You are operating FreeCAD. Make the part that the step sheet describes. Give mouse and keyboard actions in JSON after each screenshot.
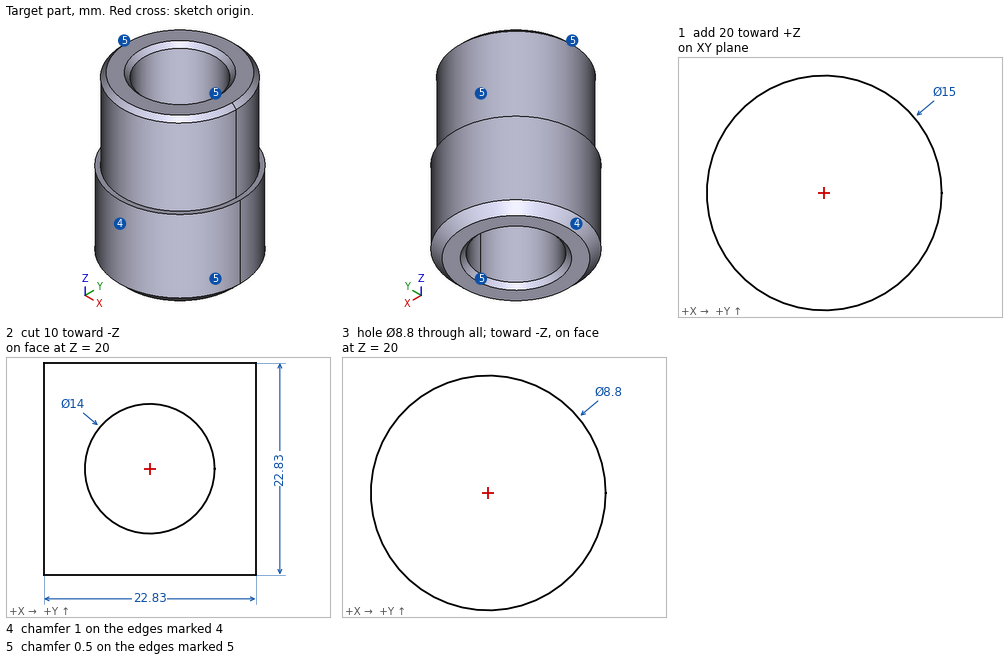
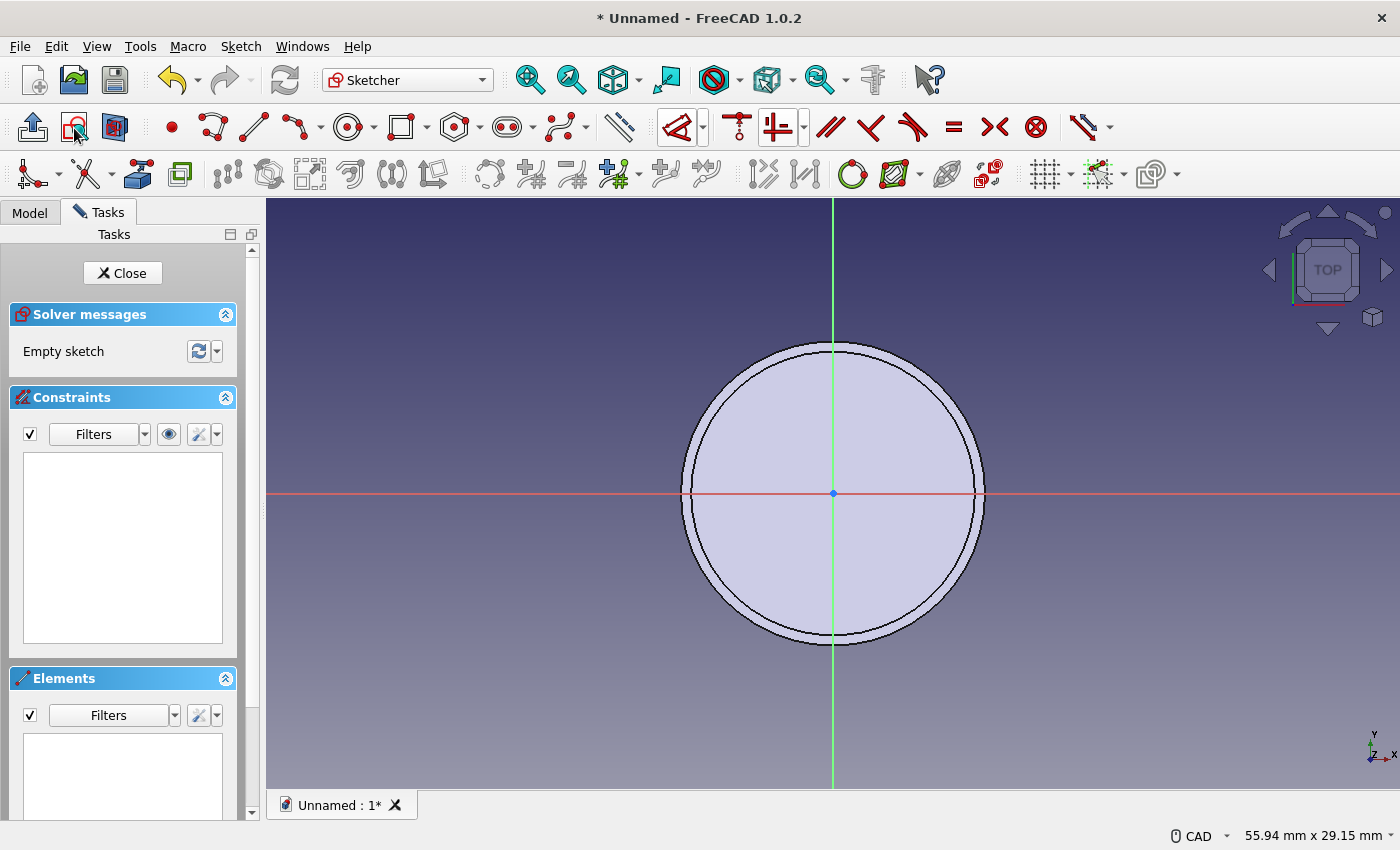
{"action": "scroll", "coordinate": [889, 494], "scroll_direction": "up", "scroll_amount": 4}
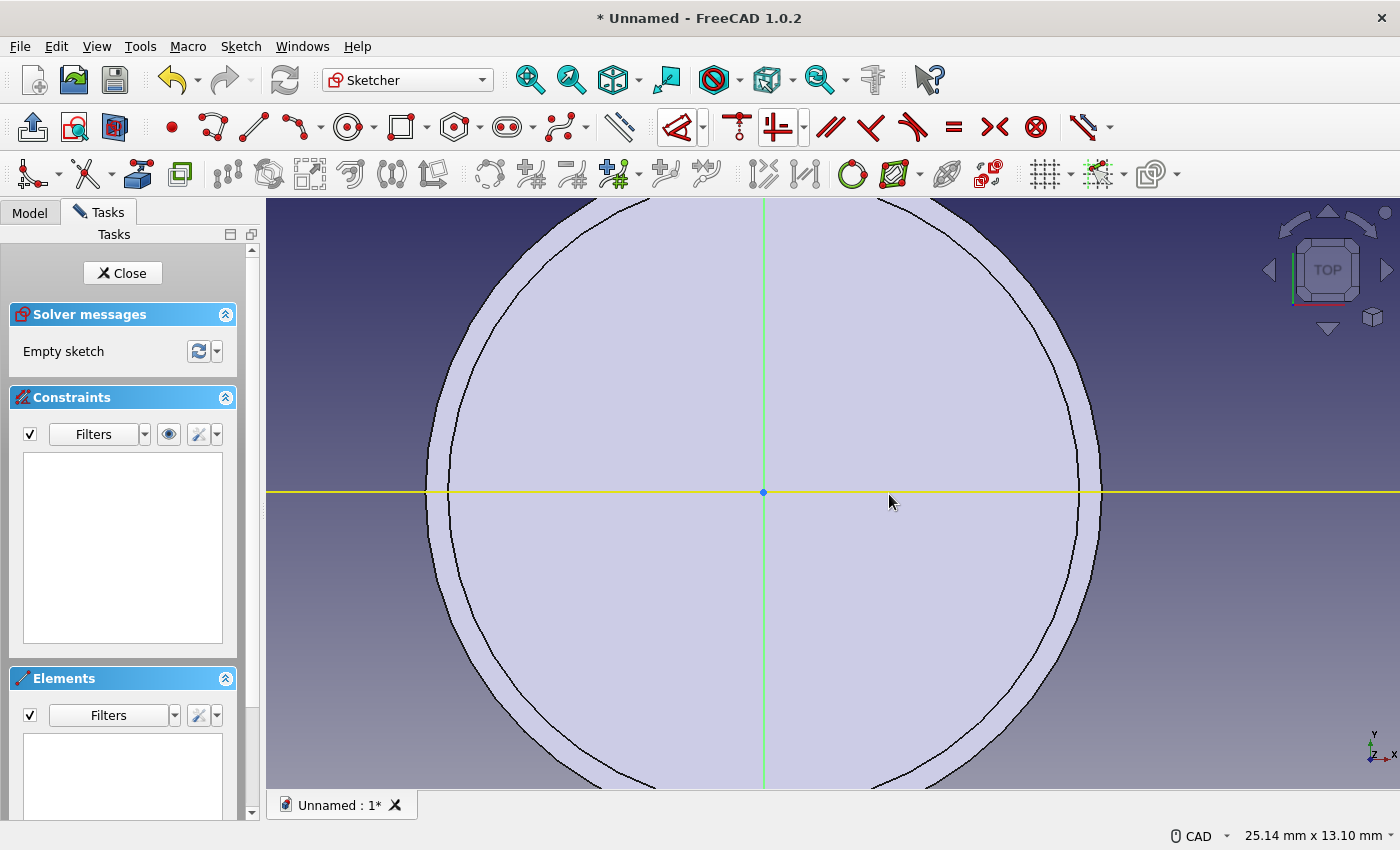
{"action": "left_click", "coordinate": [348, 128]}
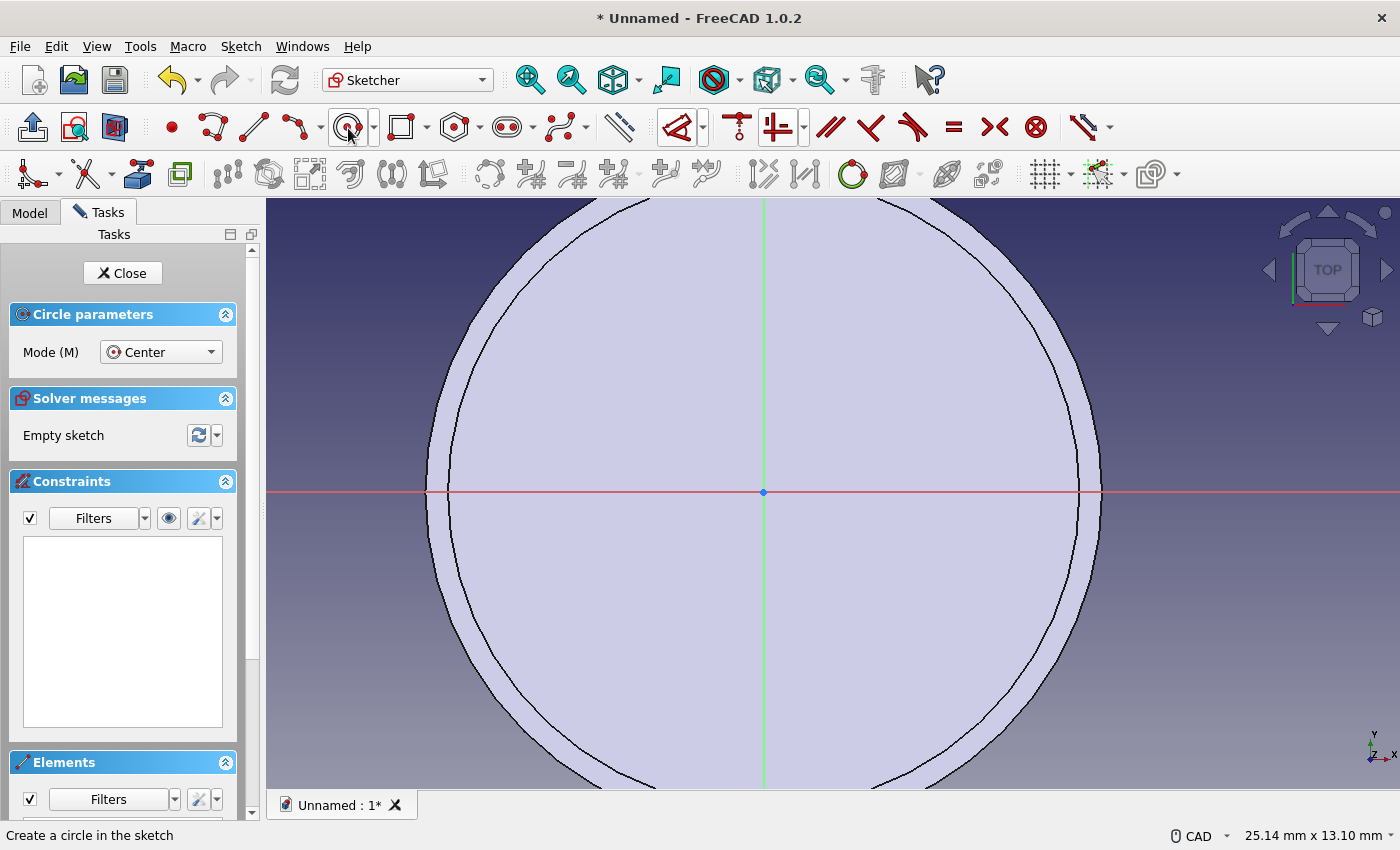
{"action": "left_click", "coordinate": [764, 492]}
{"action": "mouse_move", "coordinate": [904, 352]}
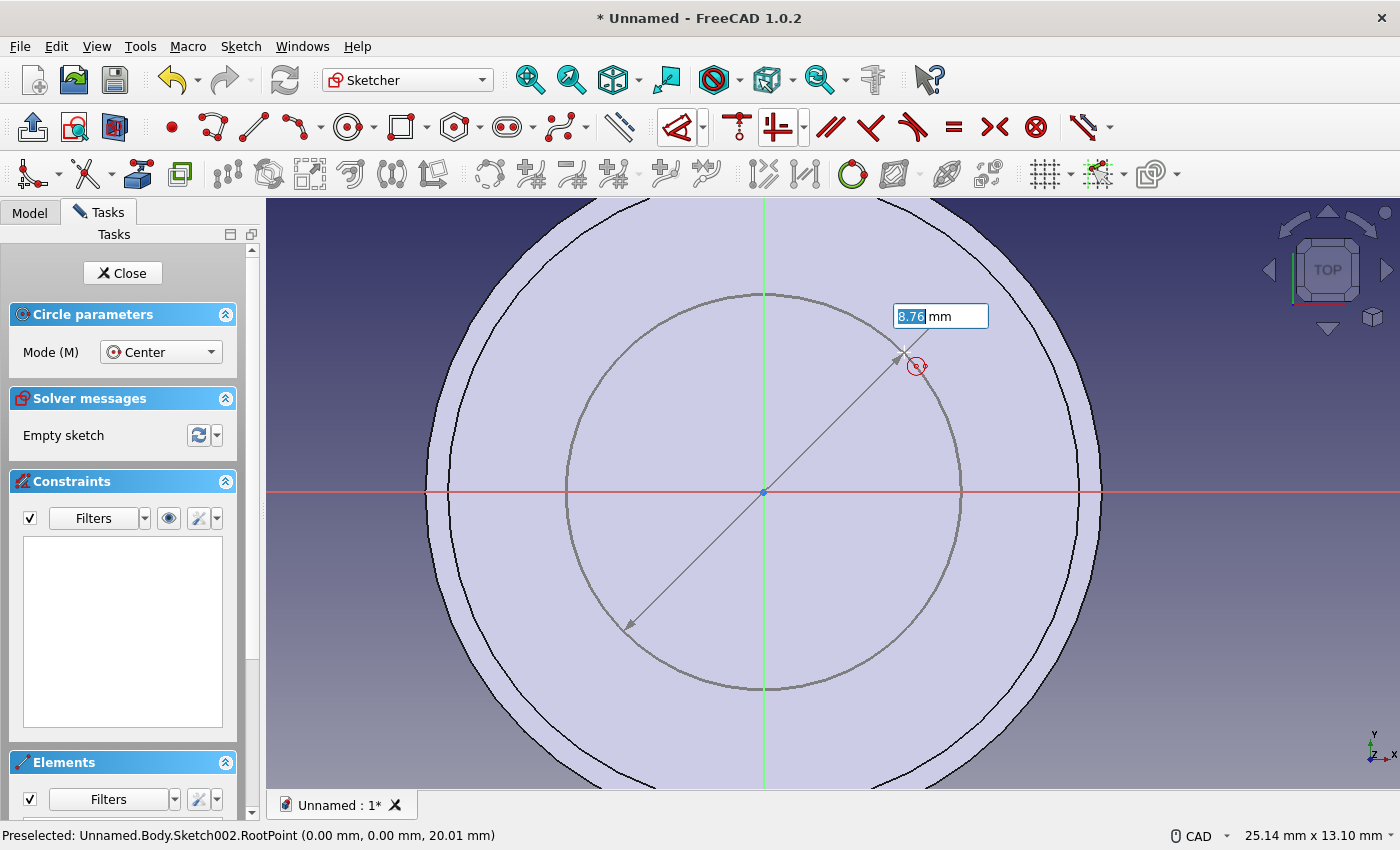
{"action": "type", "text": "8.8"}
{"action": "key", "text": "Return"}
{"action": "key", "text": "Escape"}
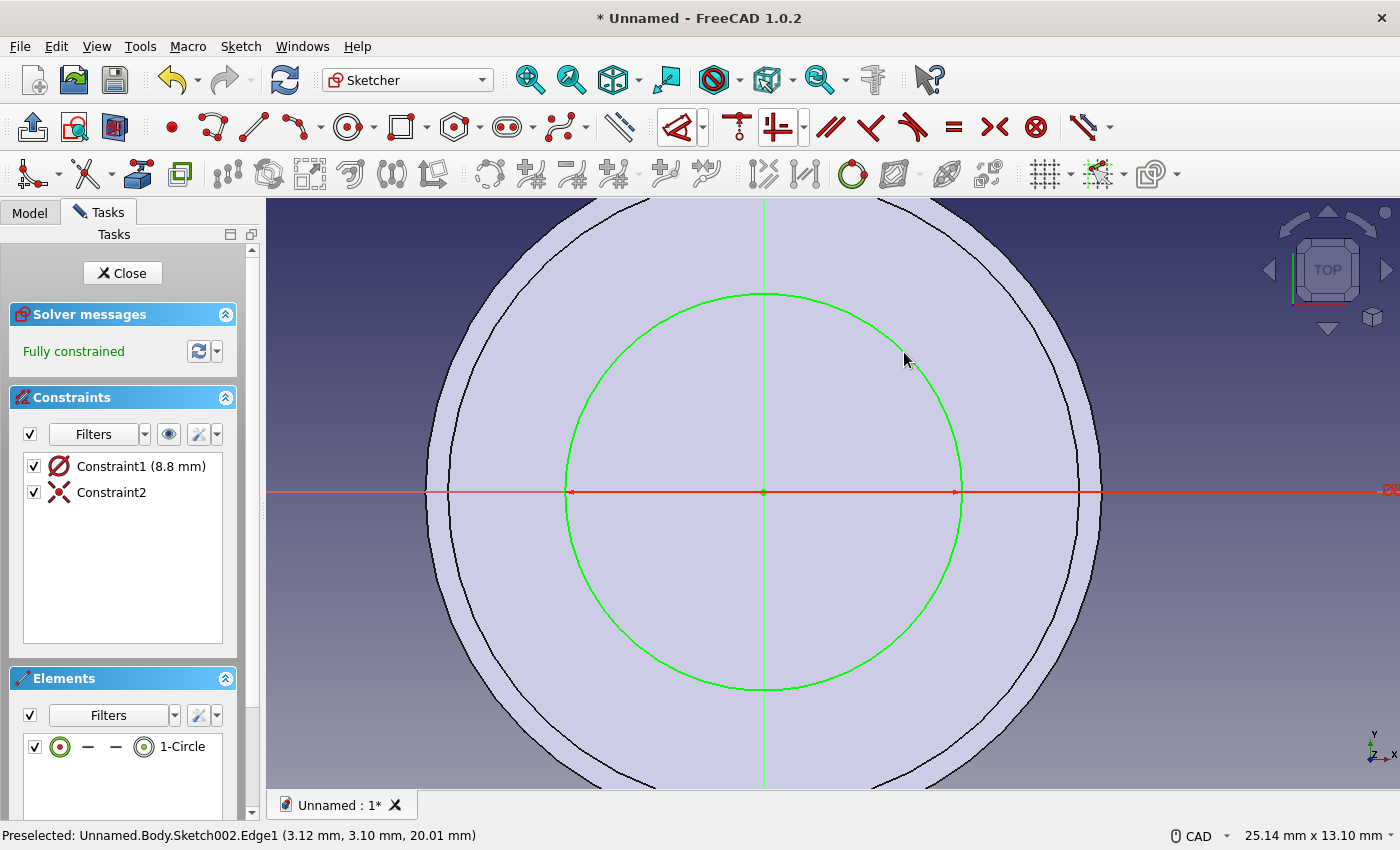
{"action": "left_click", "coordinate": [123, 273]}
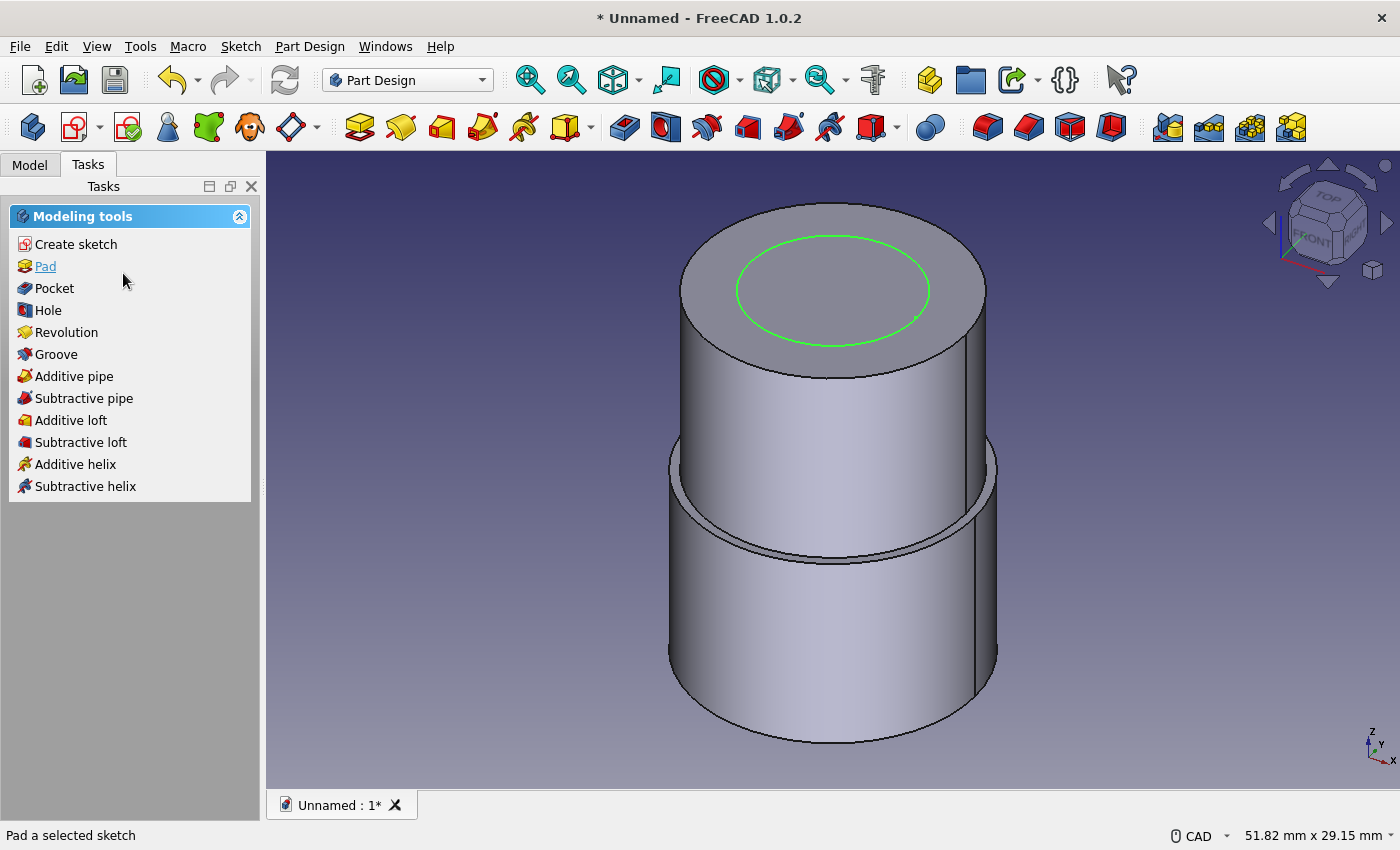
{"action": "left_click", "coordinate": [666, 128]}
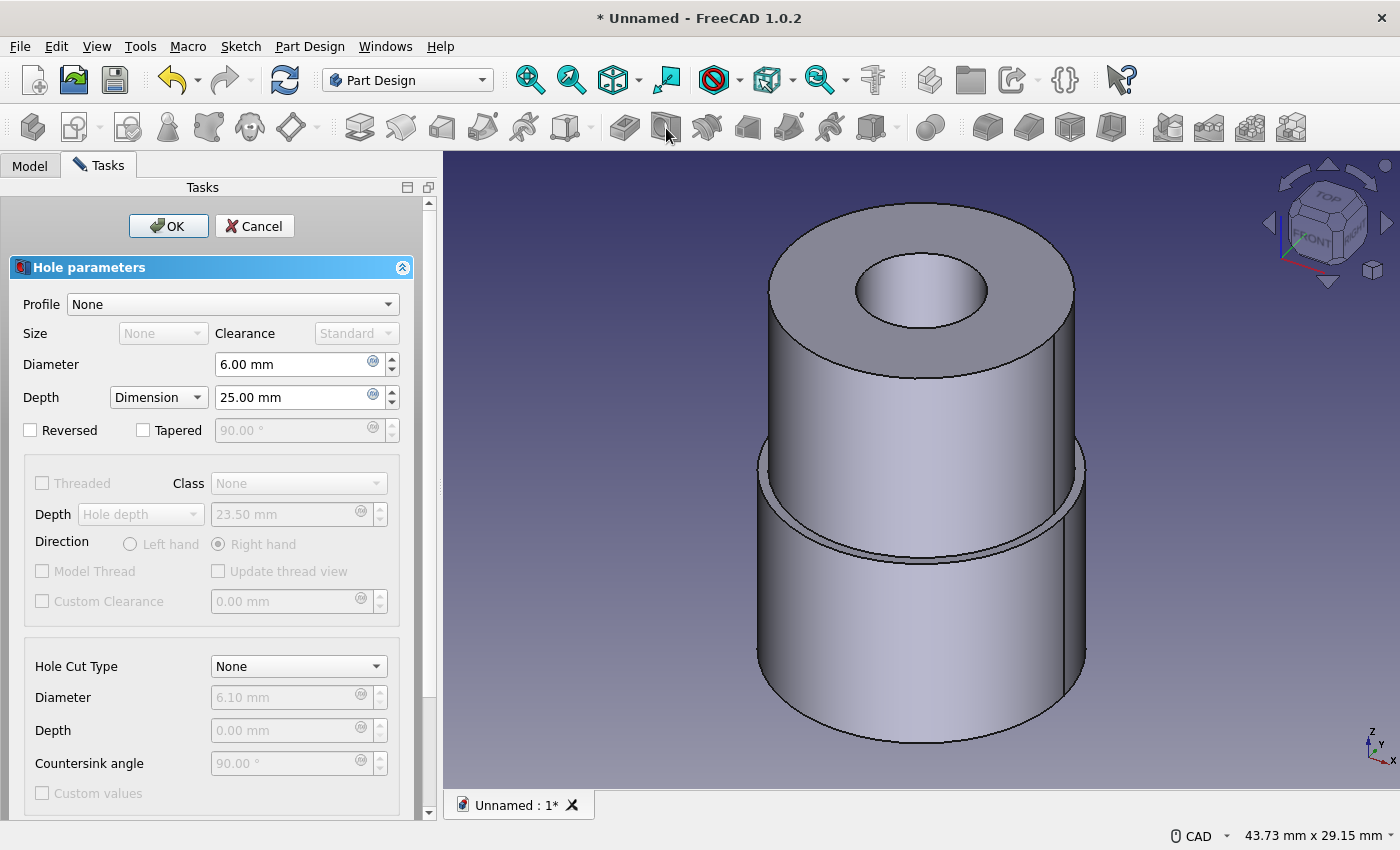
{"action": "triple_click", "coordinate": [300, 364]}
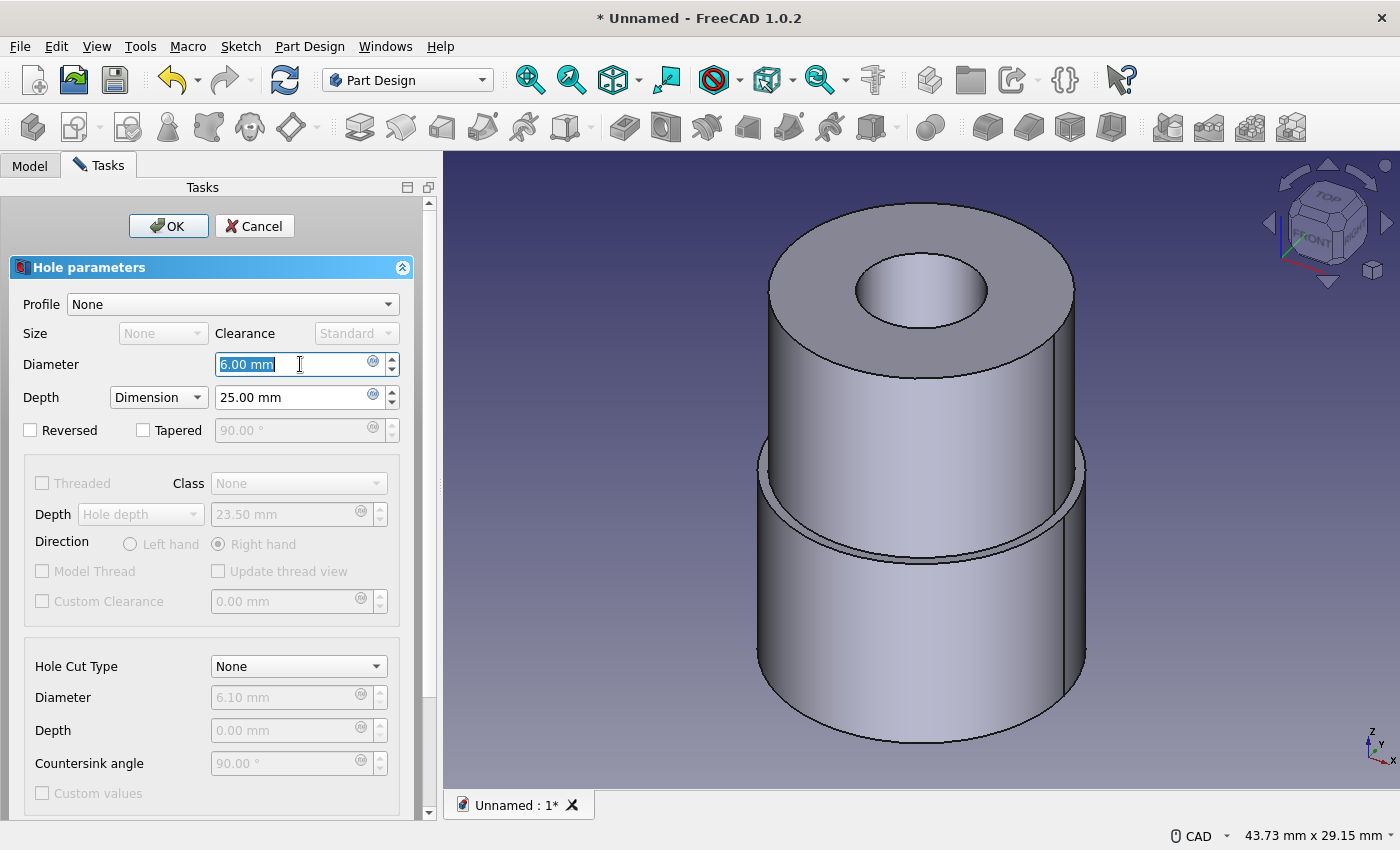
{"action": "type", "text": "8.8"}
{"action": "key", "text": "Tab"}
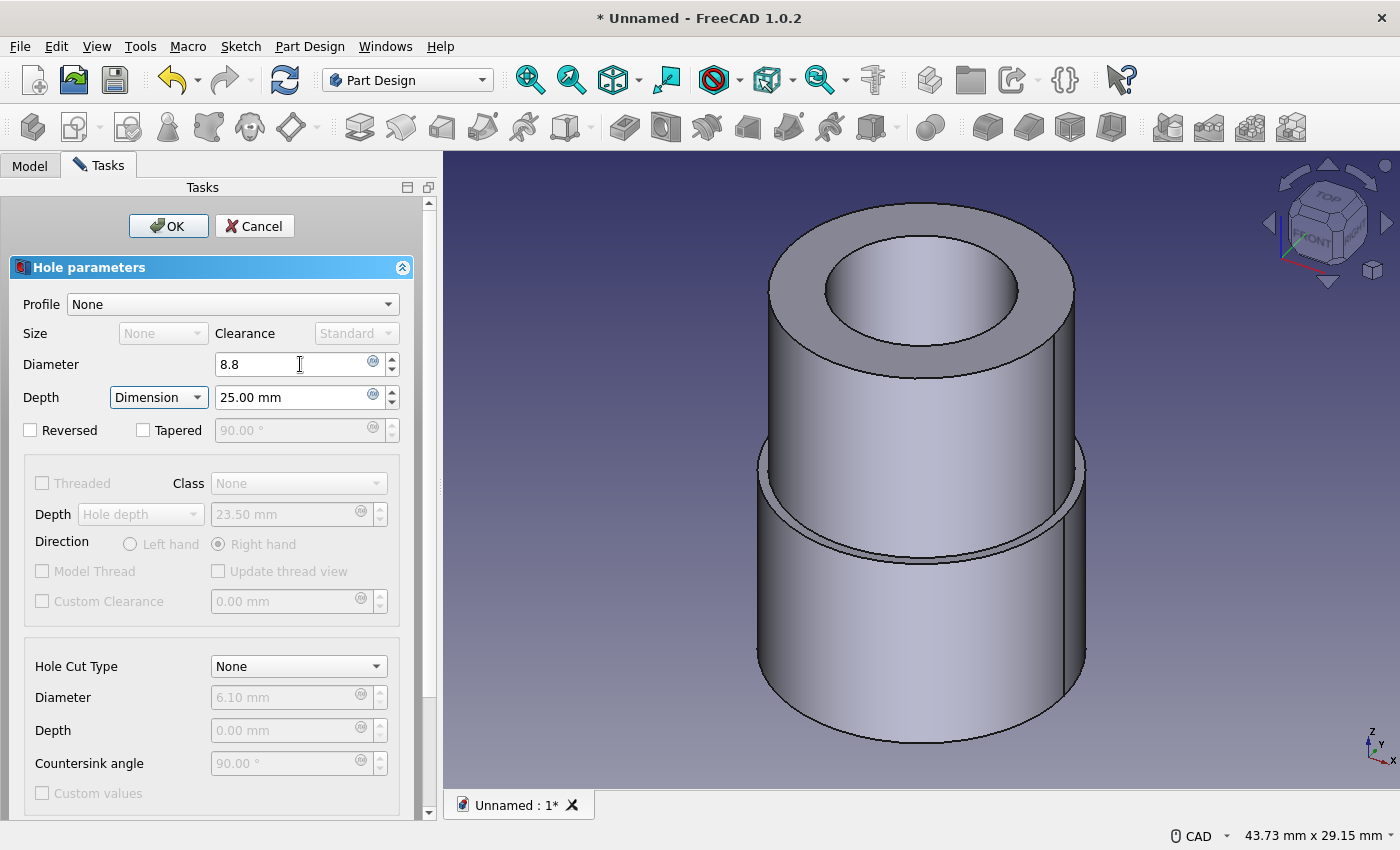
{"action": "left_click", "coordinate": [160, 398]}